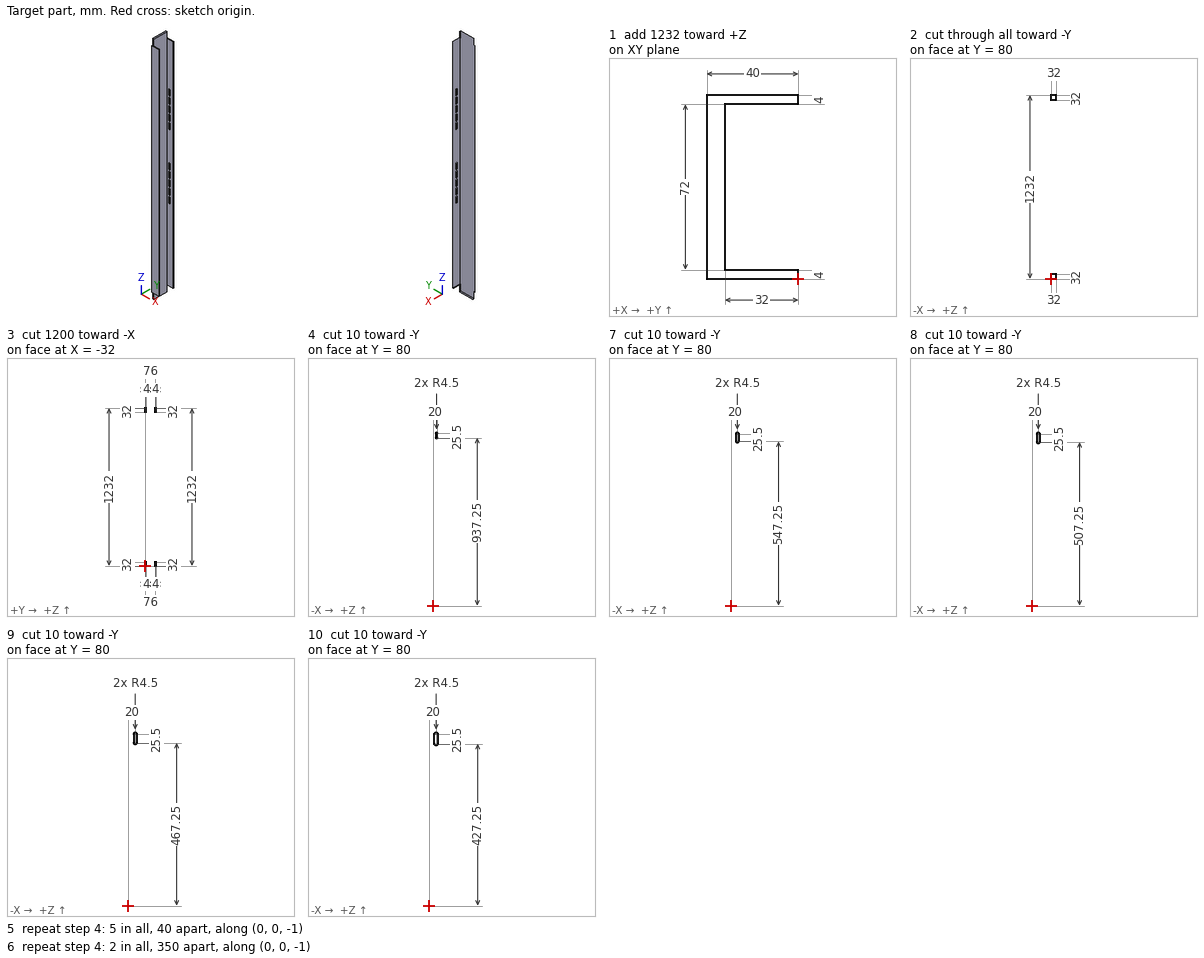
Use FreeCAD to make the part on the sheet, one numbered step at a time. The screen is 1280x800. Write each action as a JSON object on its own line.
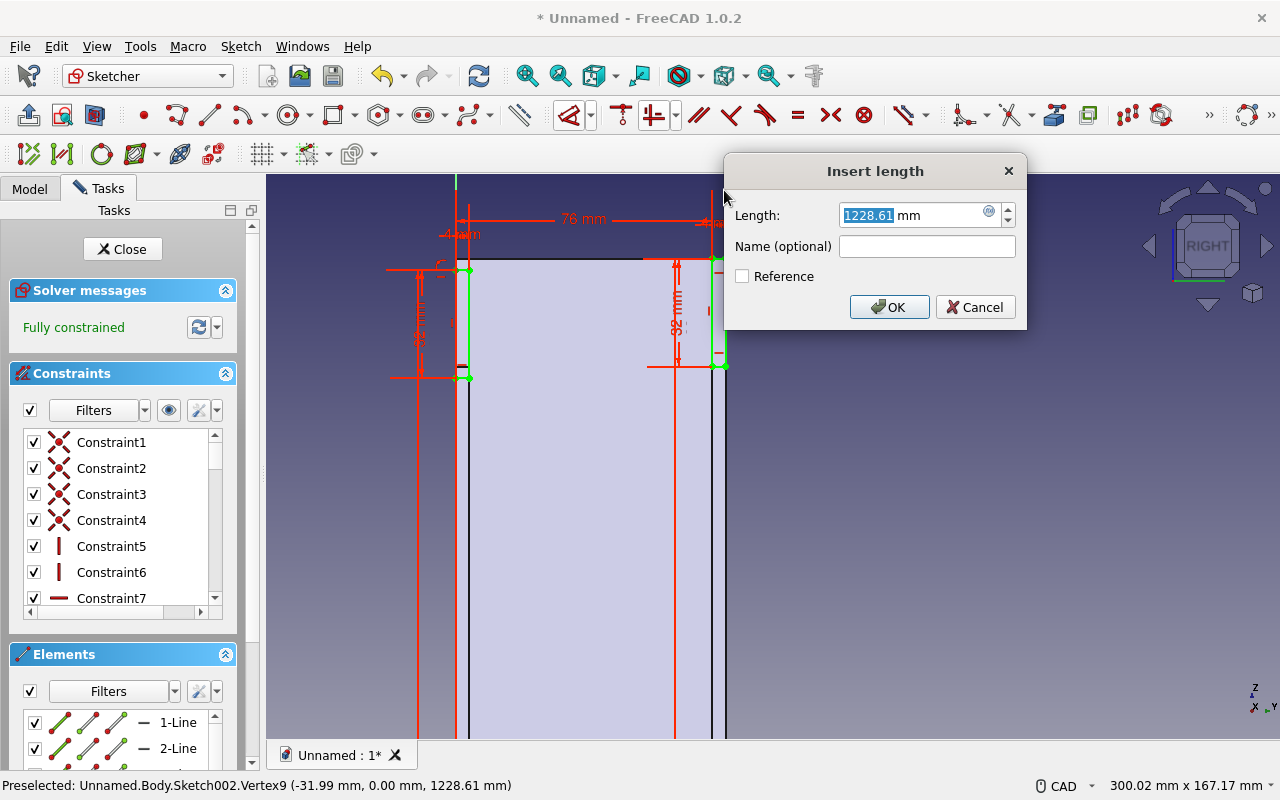
{"action": "type", "text": "1232"}
{"action": "key", "text": "Return"}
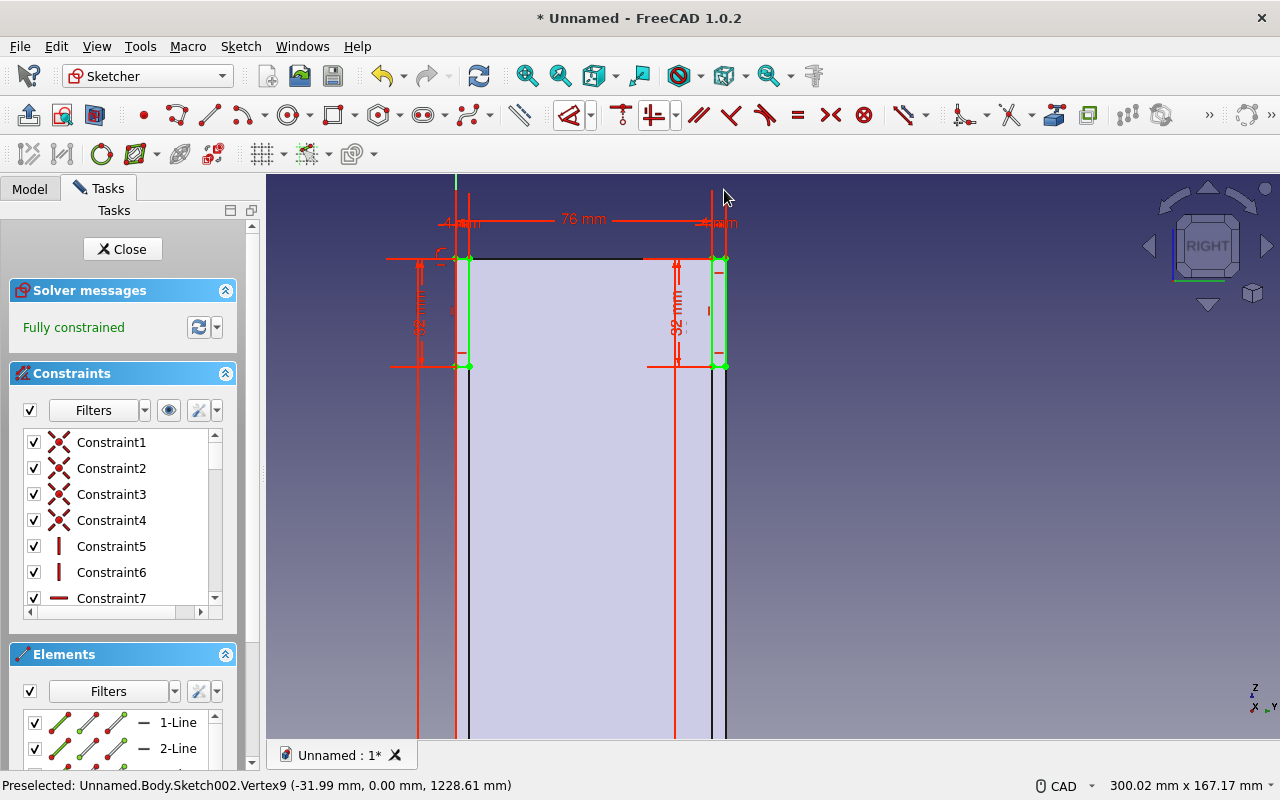
{"action": "left_click", "coordinate": [123, 249]}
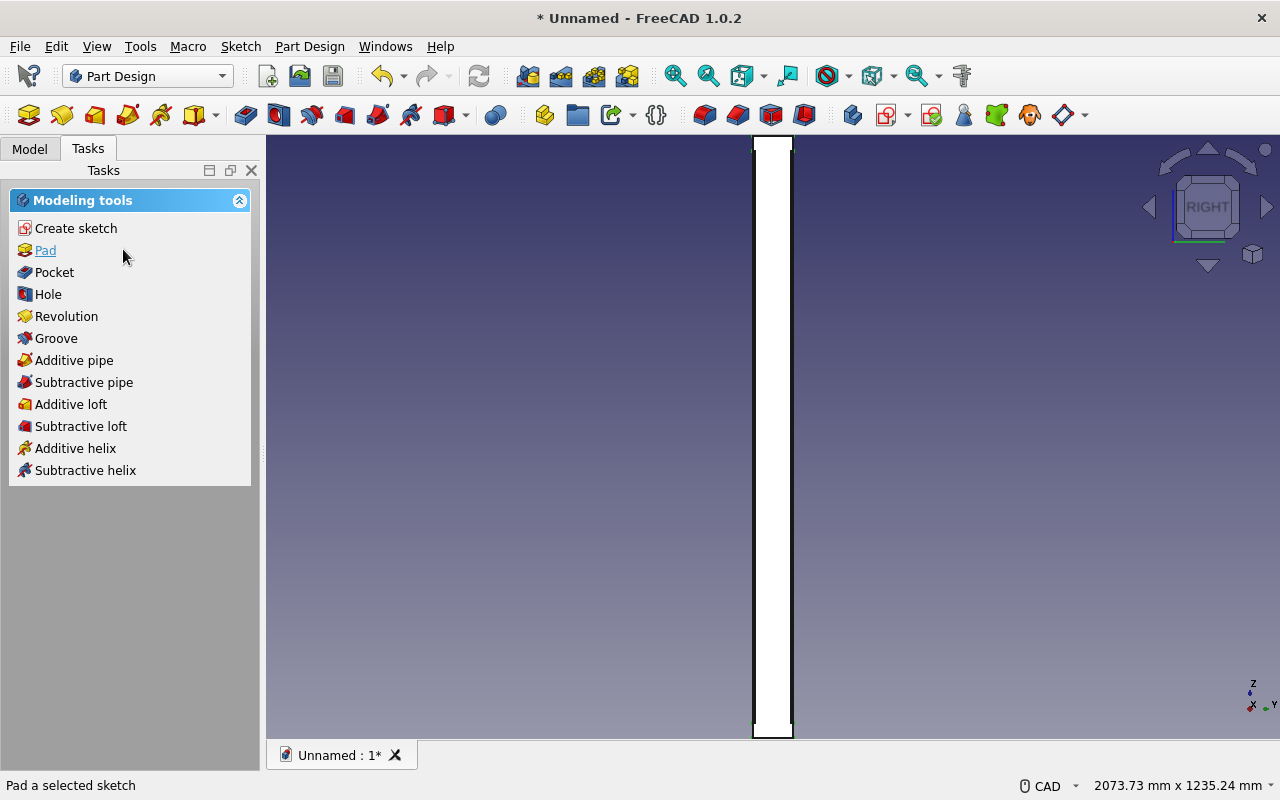
{"action": "left_click", "coordinate": [246, 116]}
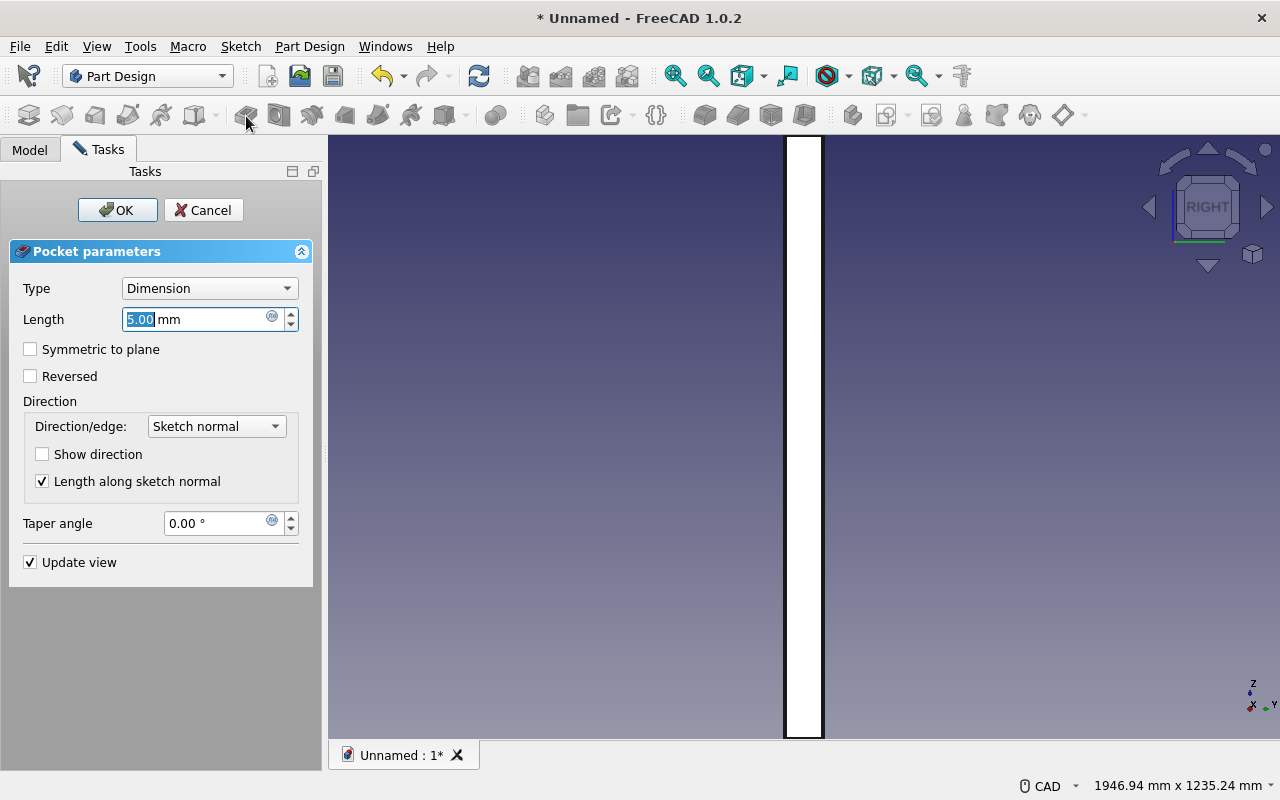
{"action": "type", "text": "1200"}
{"action": "key", "text": "Tab"}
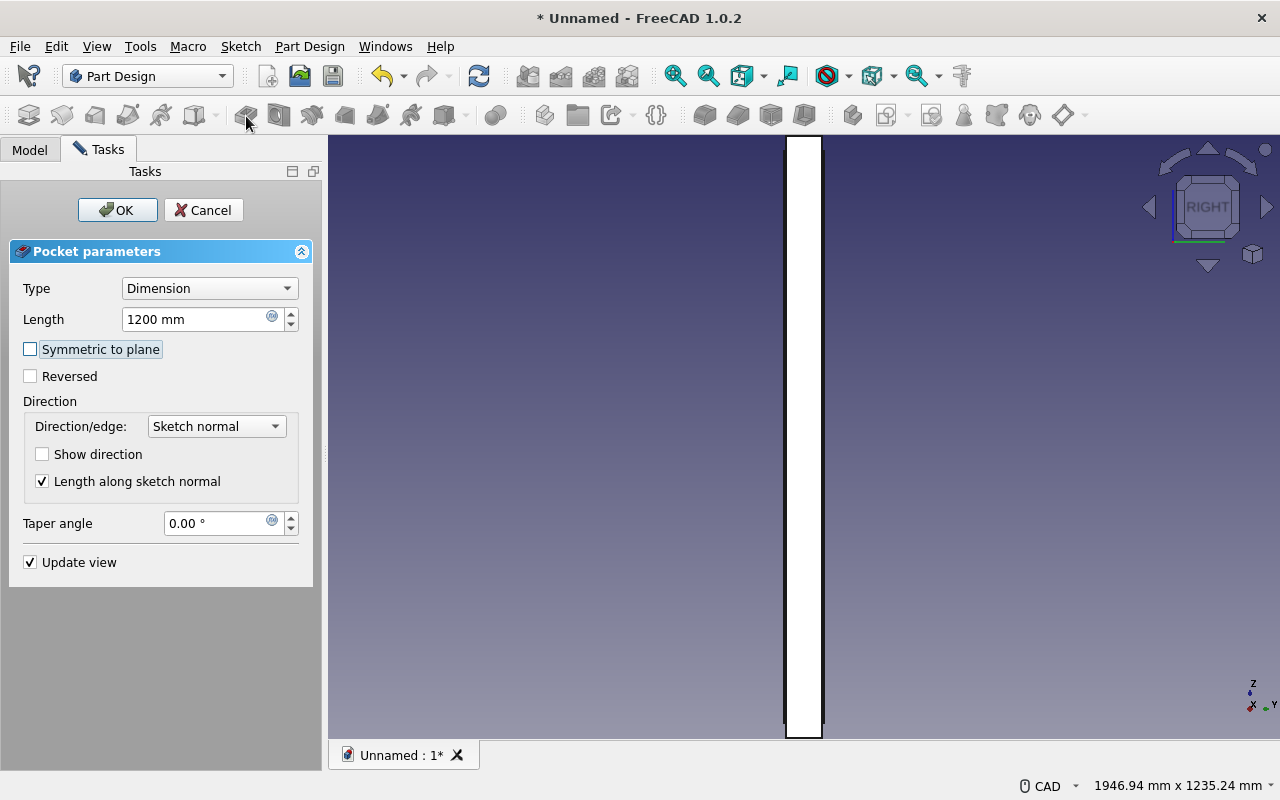
{"action": "left_click", "coordinate": [118, 210]}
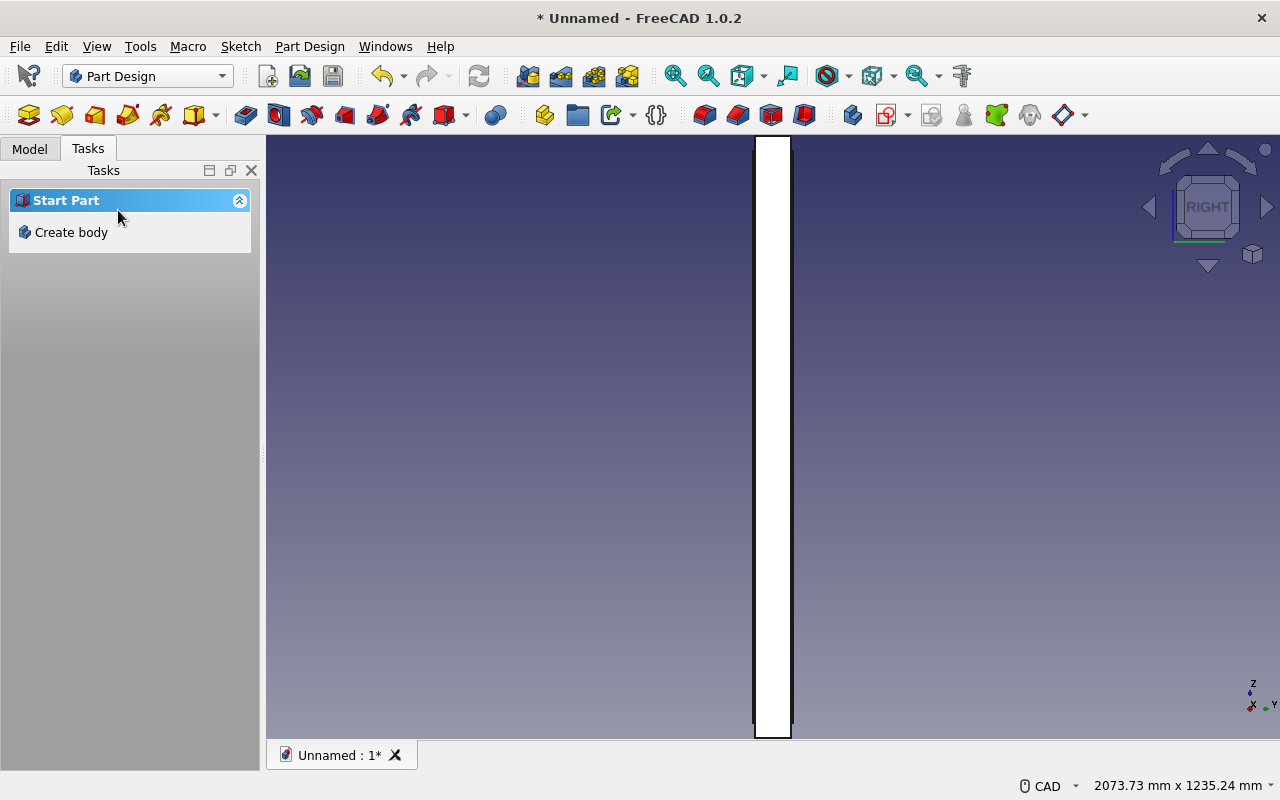
{"action": "key", "text": "4"}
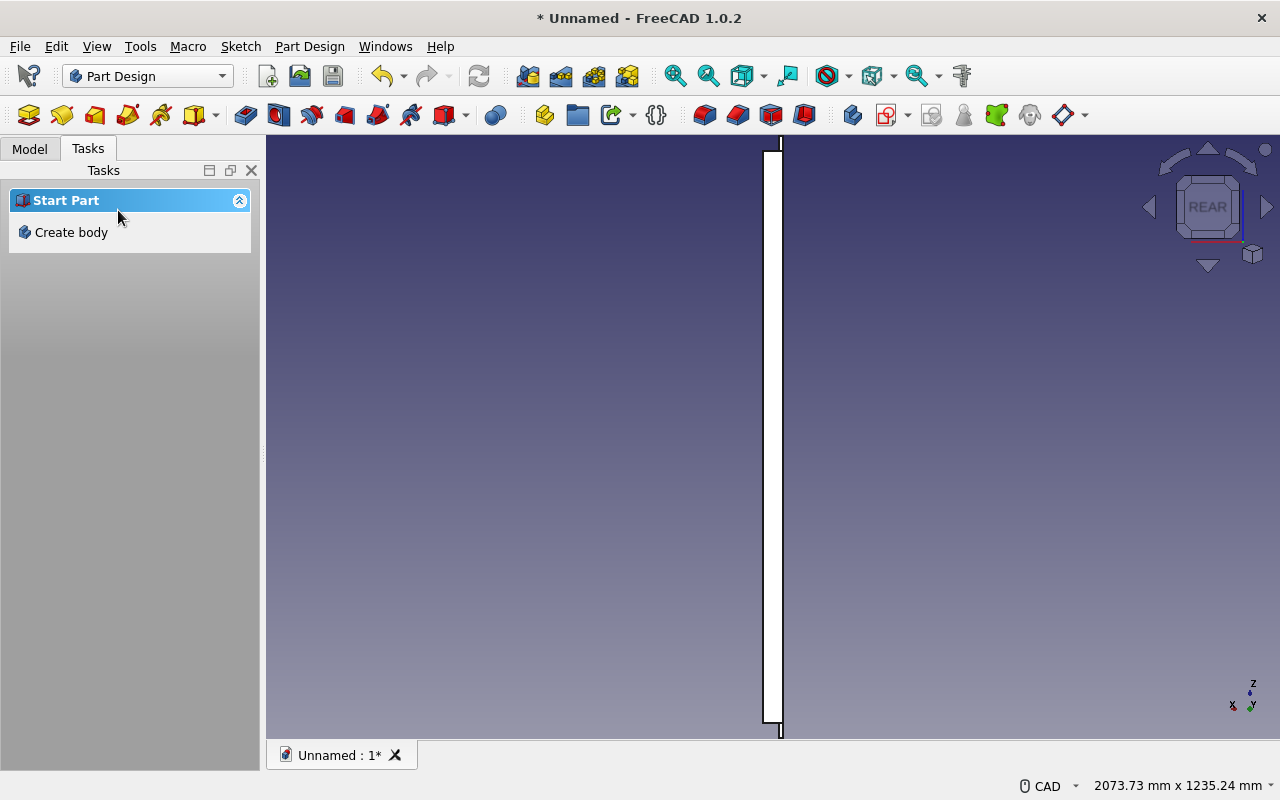
{"action": "left_click", "coordinate": [773, 191]}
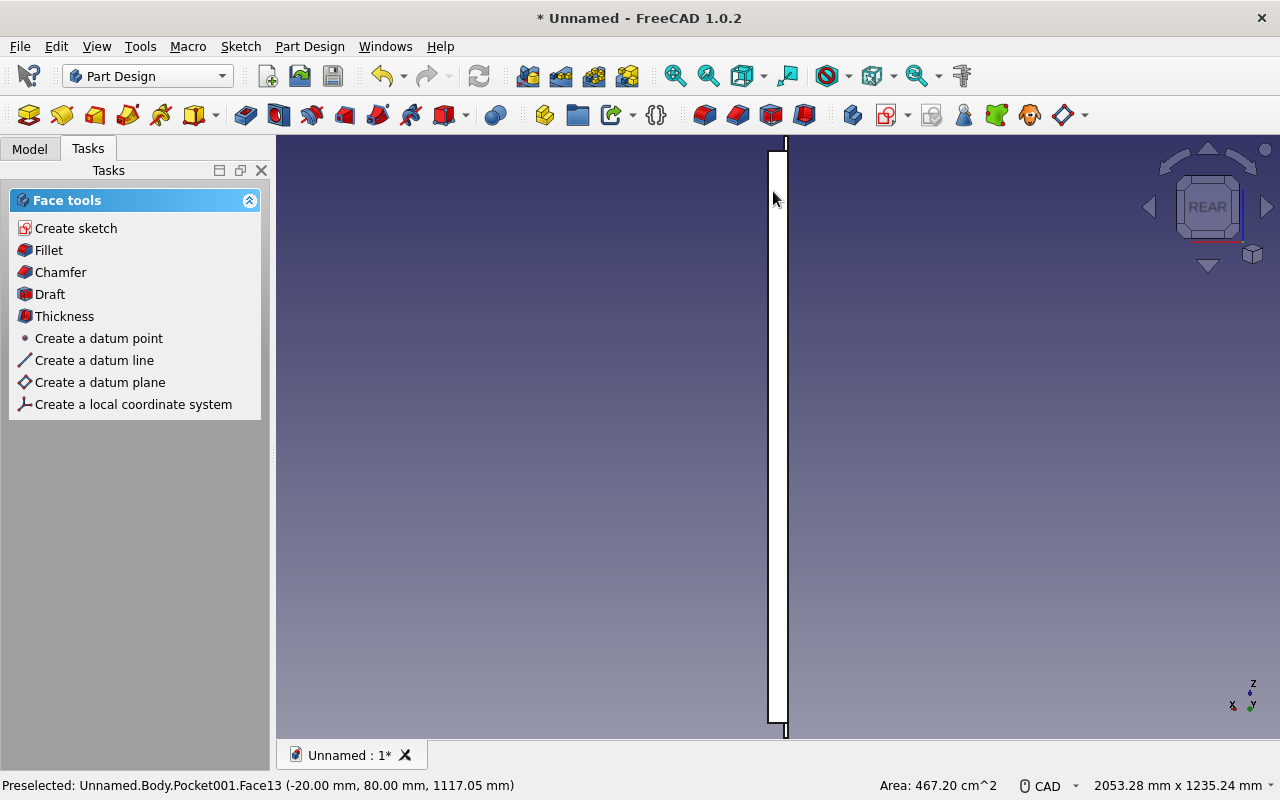
{"action": "left_click", "coordinate": [886, 116]}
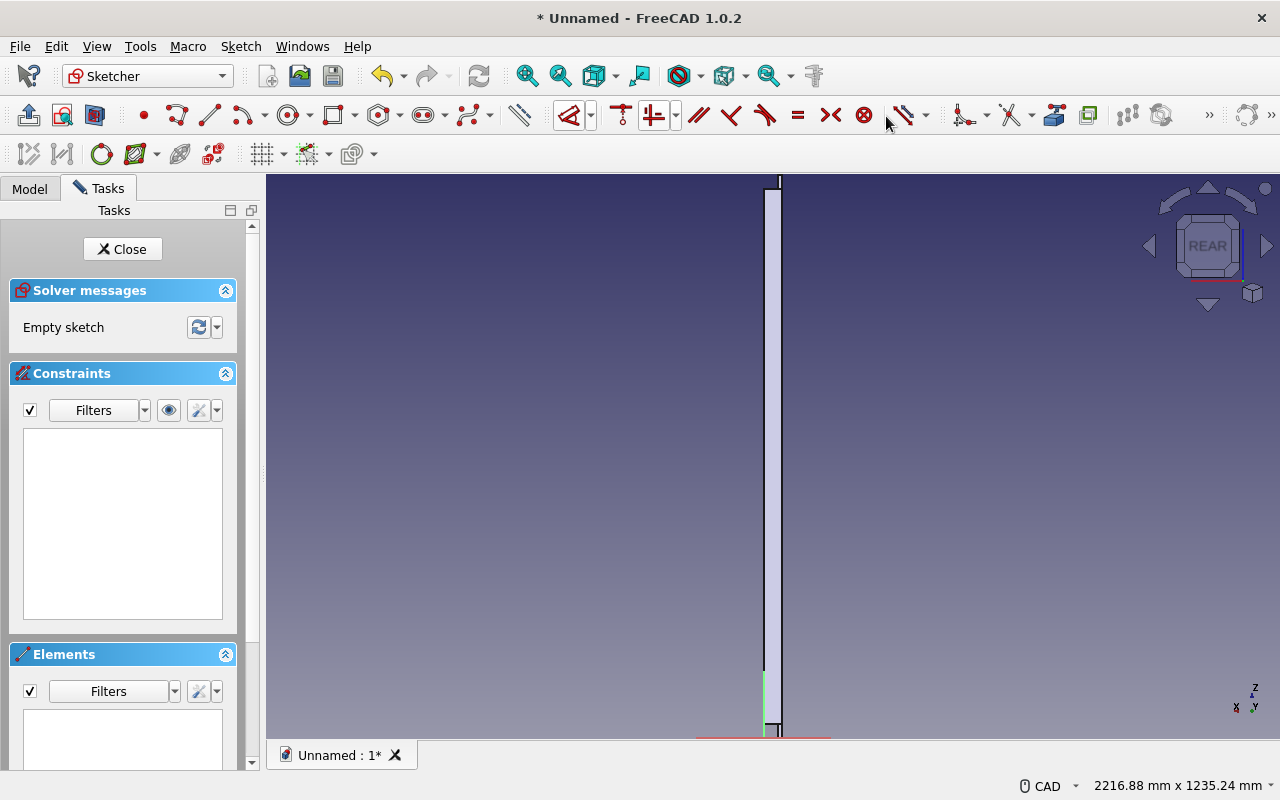
{"action": "scroll", "coordinate": [777, 296], "scroll_direction": "up", "scroll_amount": 15}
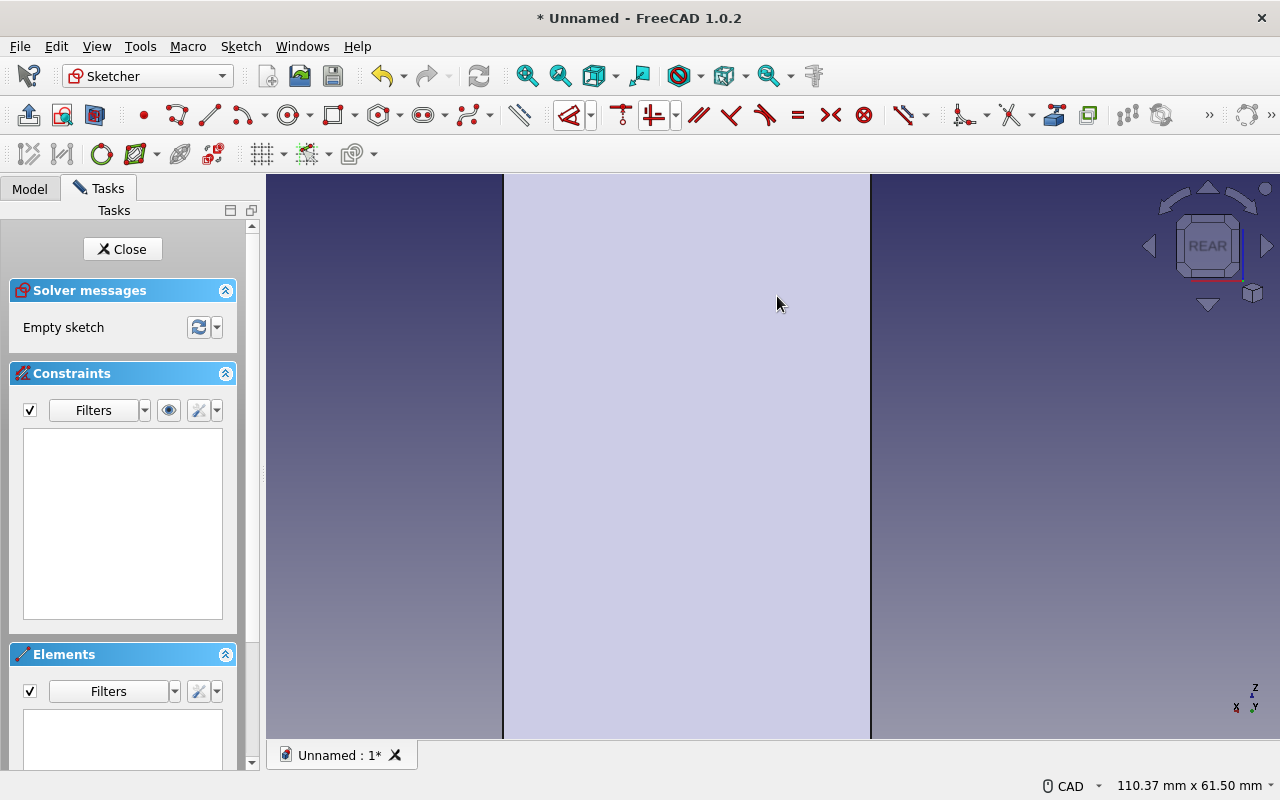
{"action": "left_click", "coordinate": [422, 116]}